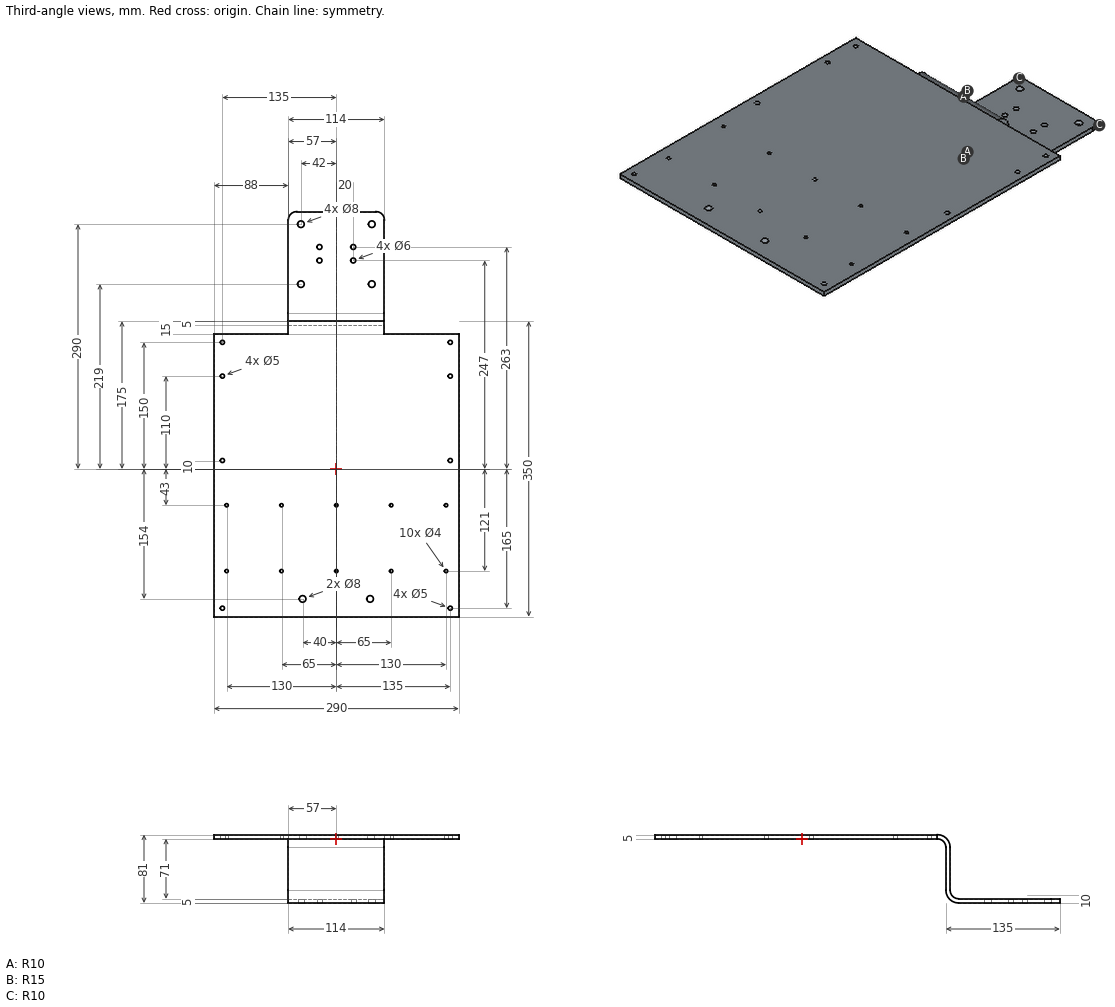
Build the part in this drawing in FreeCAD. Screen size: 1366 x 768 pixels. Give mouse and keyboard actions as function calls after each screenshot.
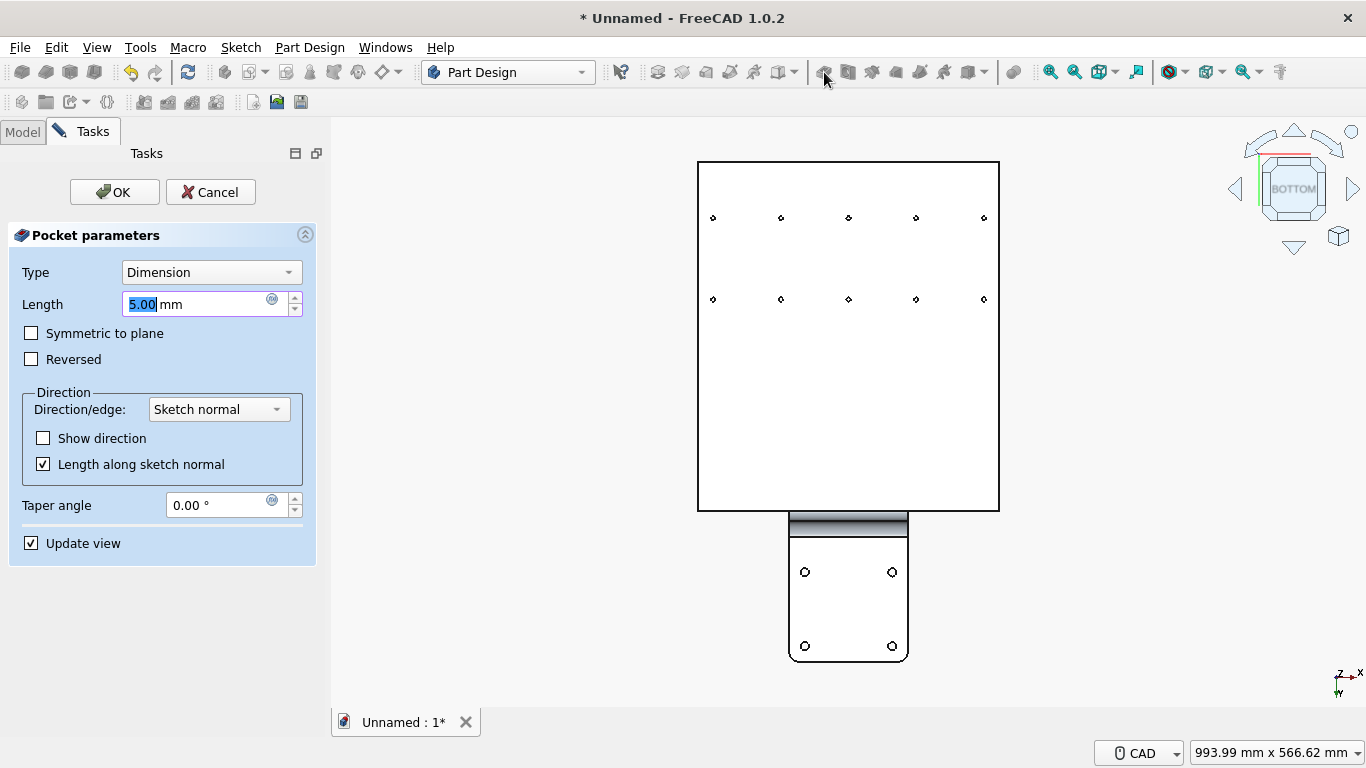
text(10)
key(Tab)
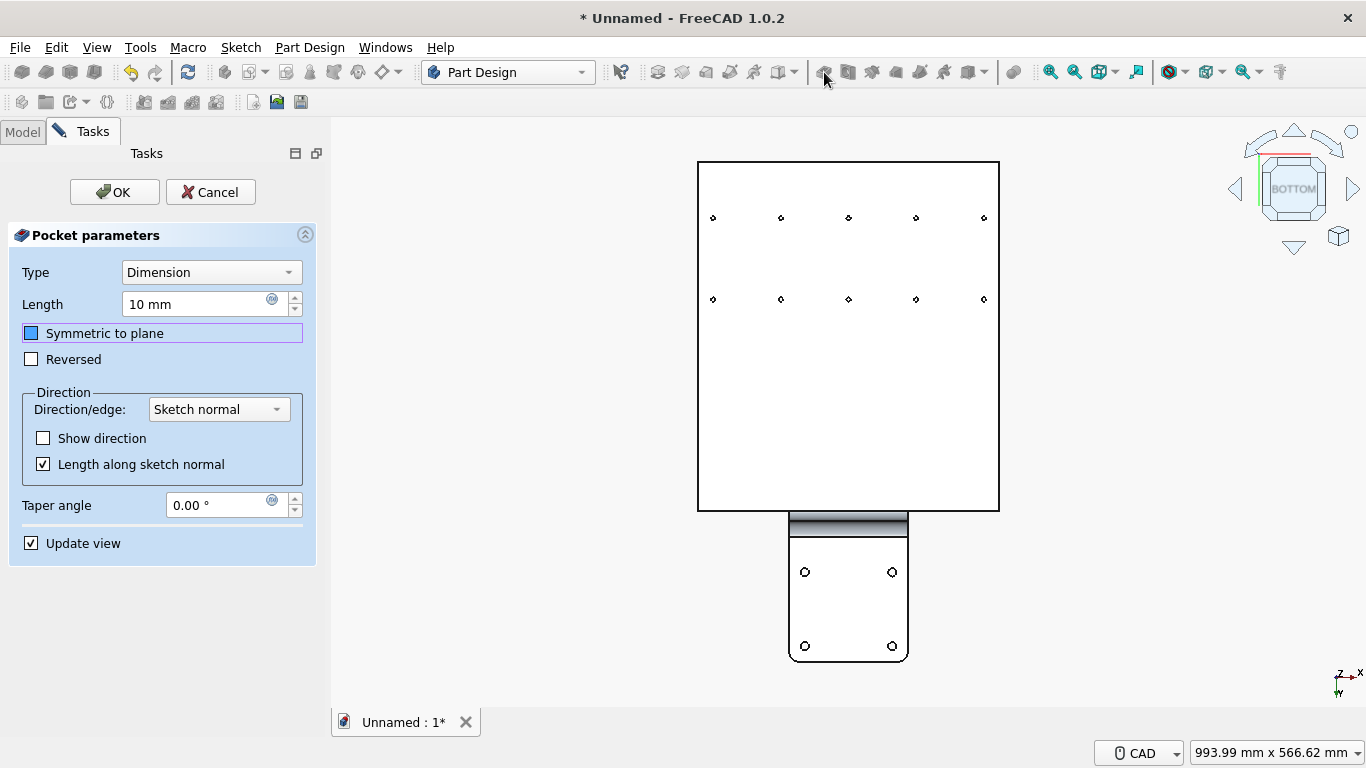
click(115, 192)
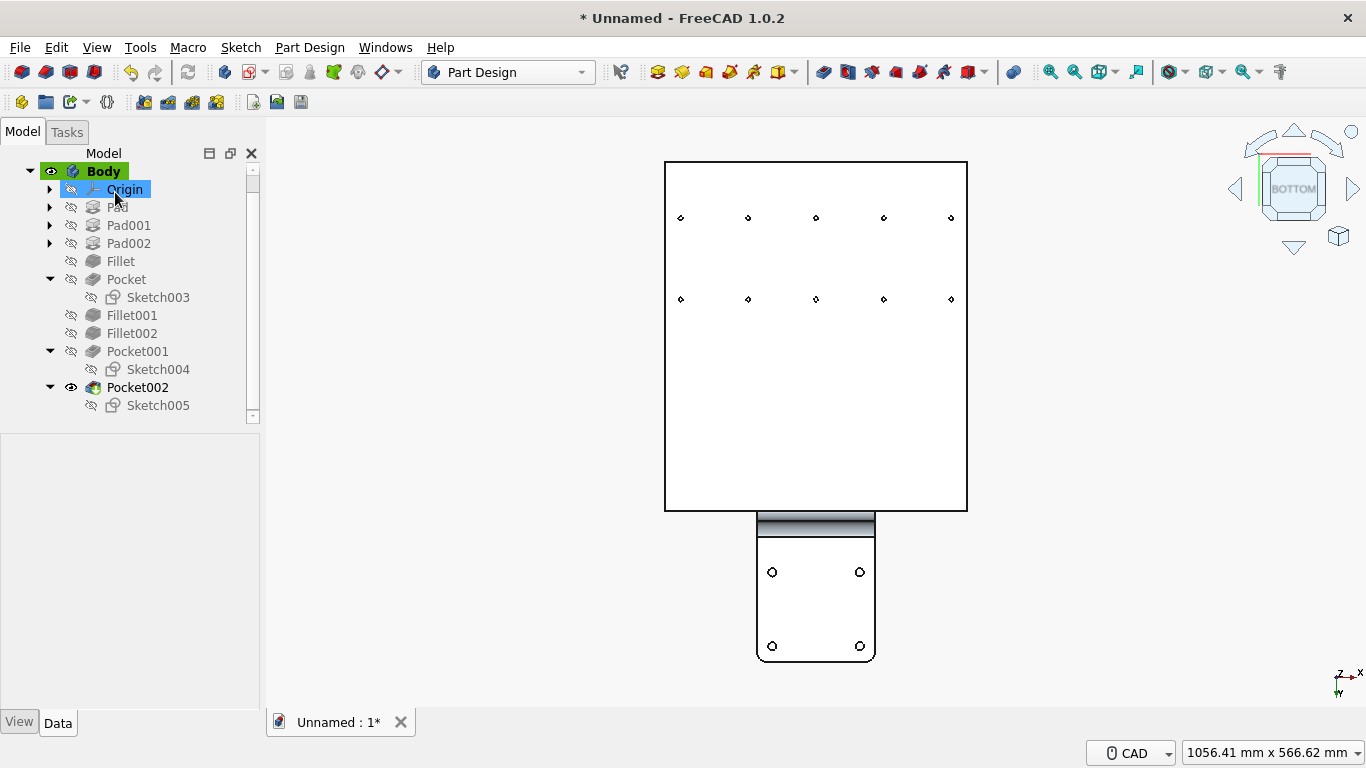
click(816, 598)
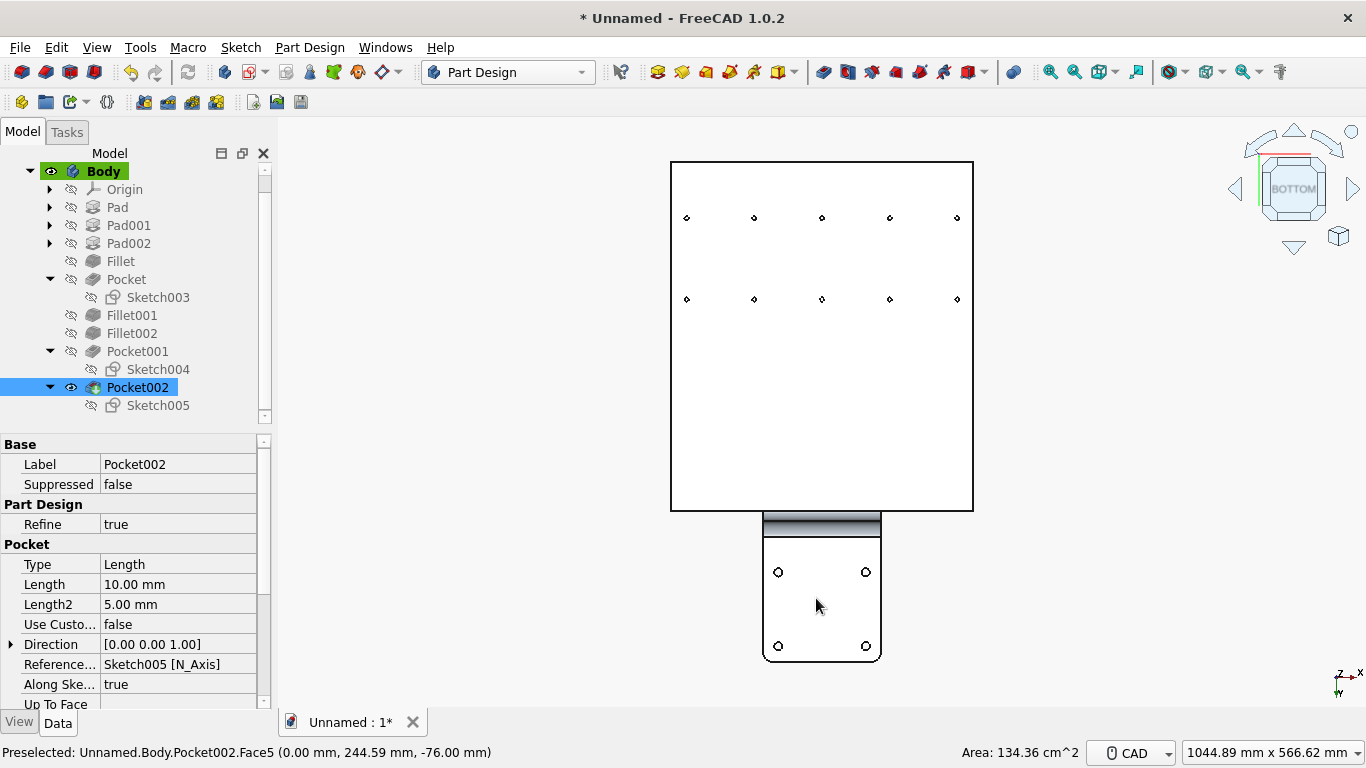
click(250, 72)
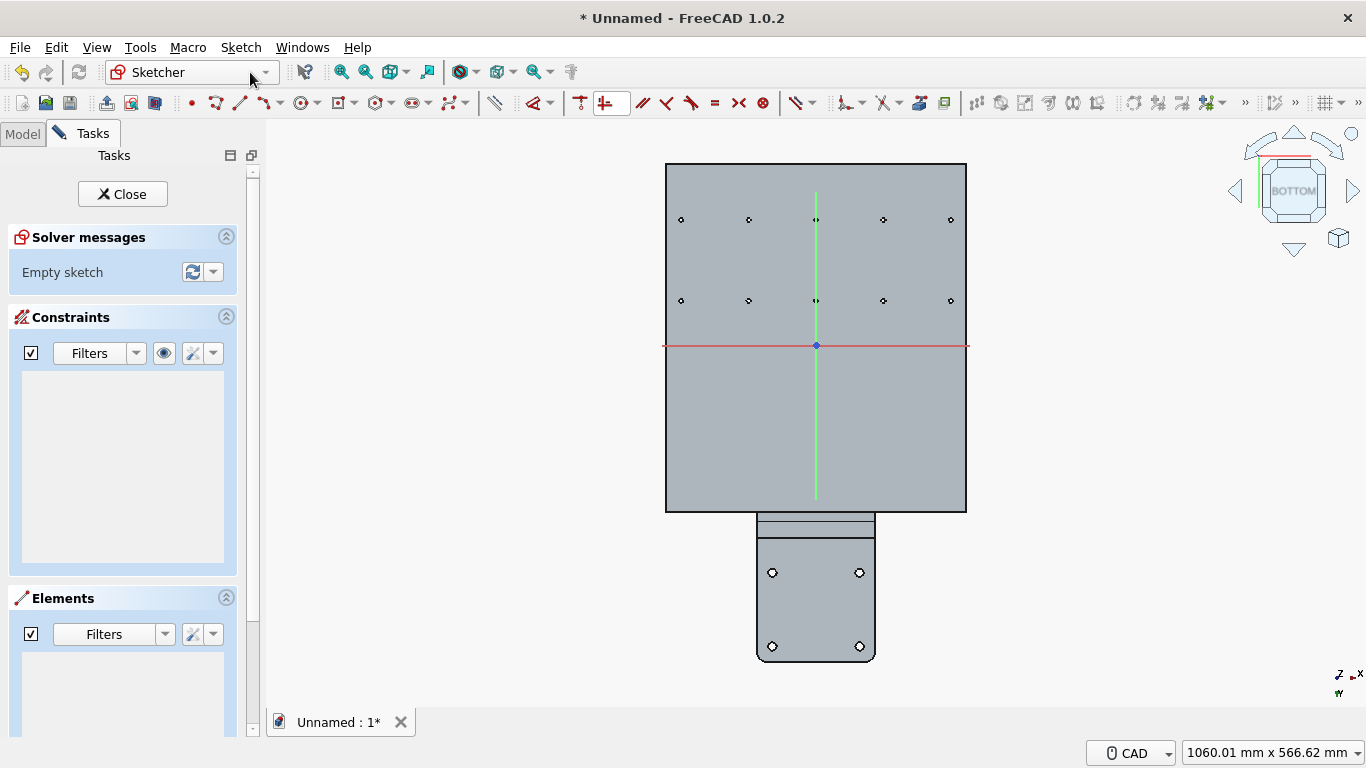
scroll(821, 626, up, 13)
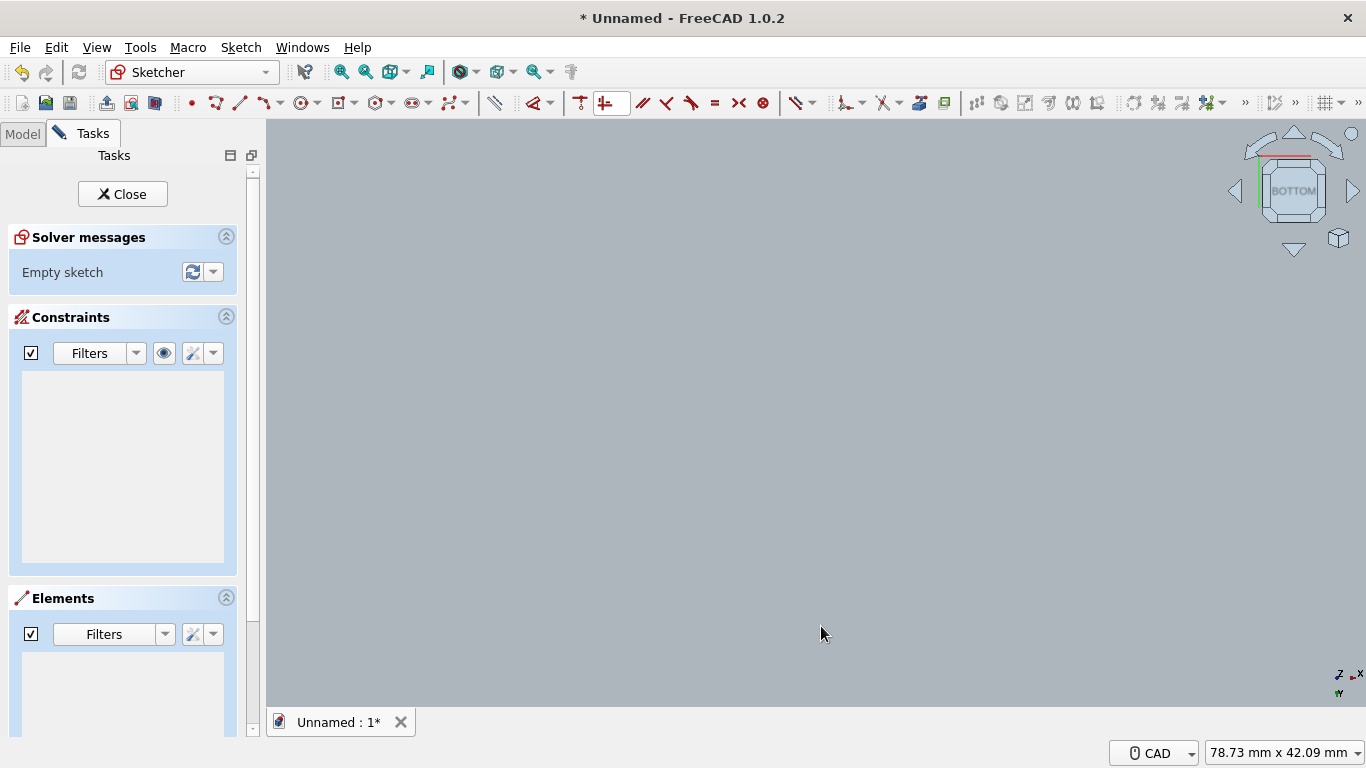
key(g)
key(c)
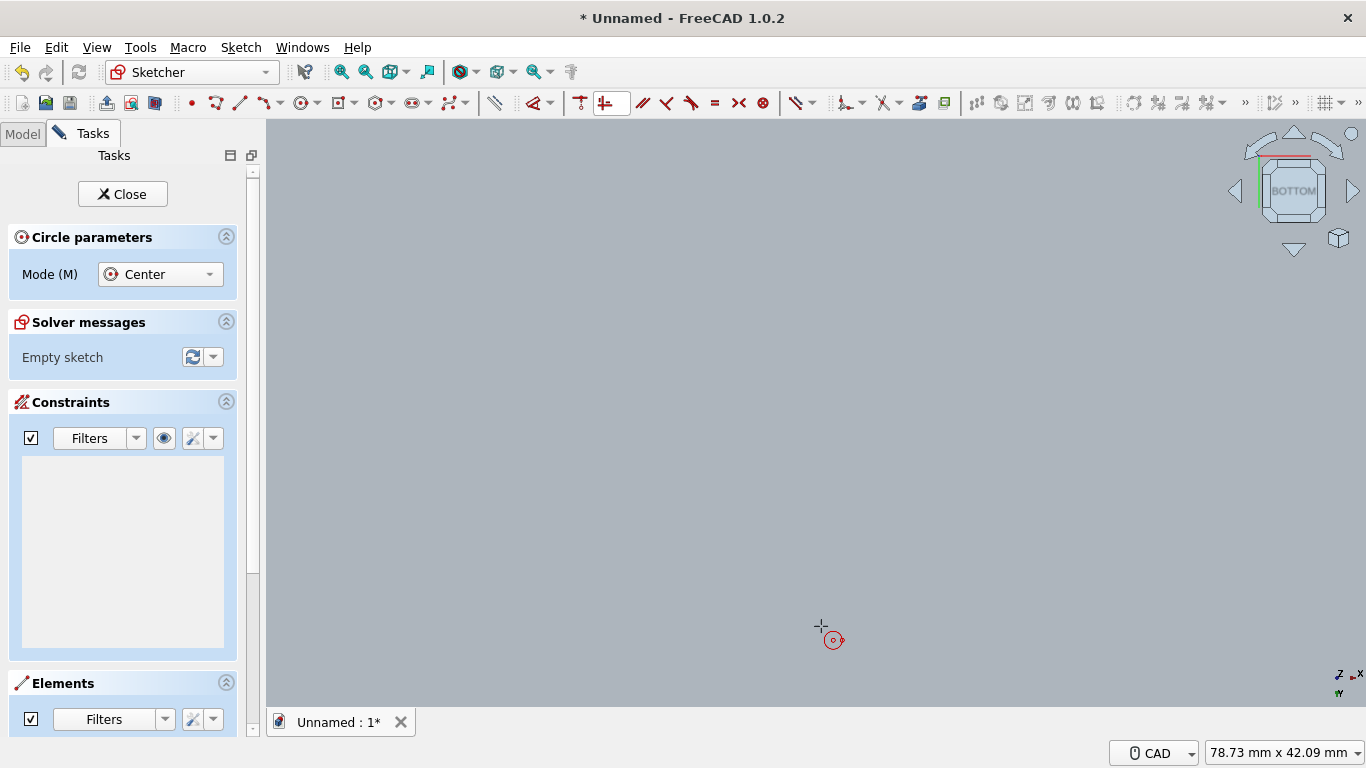
click(1027, 290)
click(1056, 261)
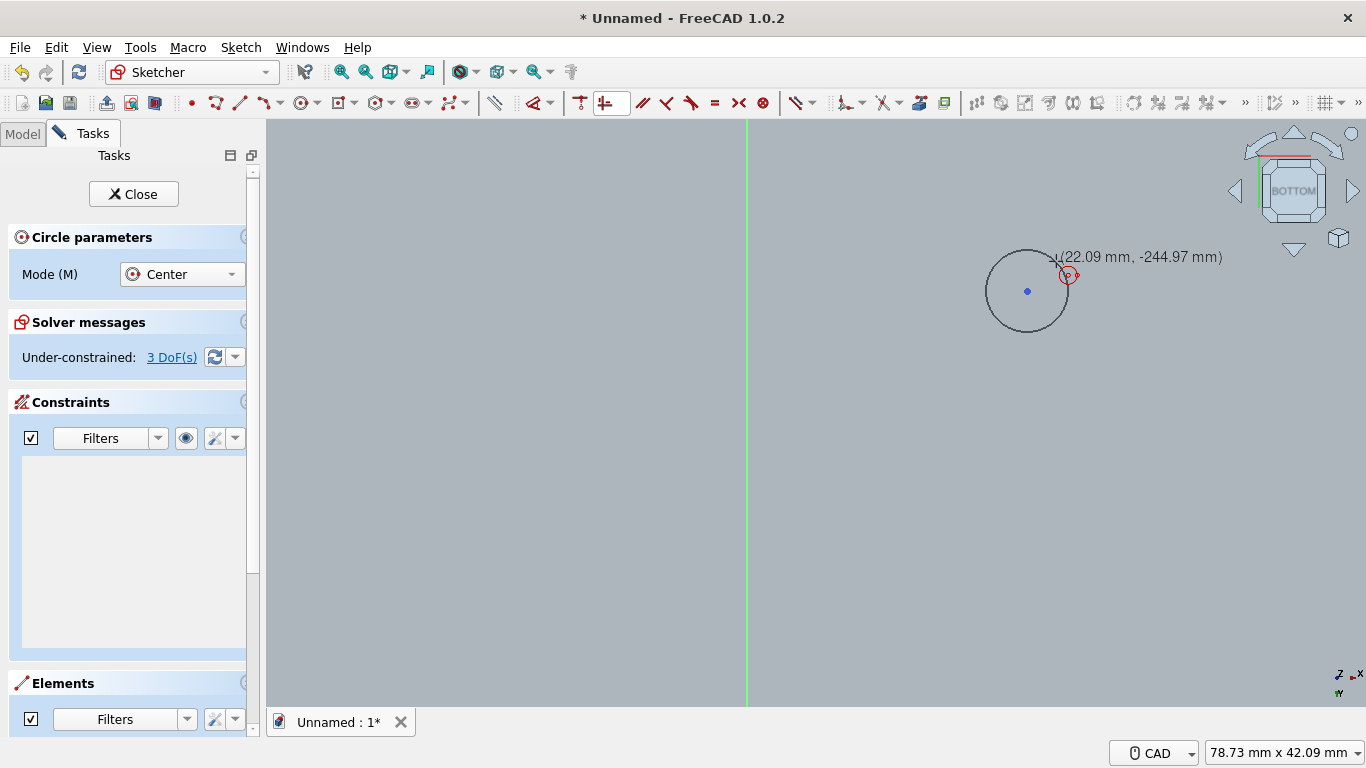
click(1027, 514)
click(1056, 484)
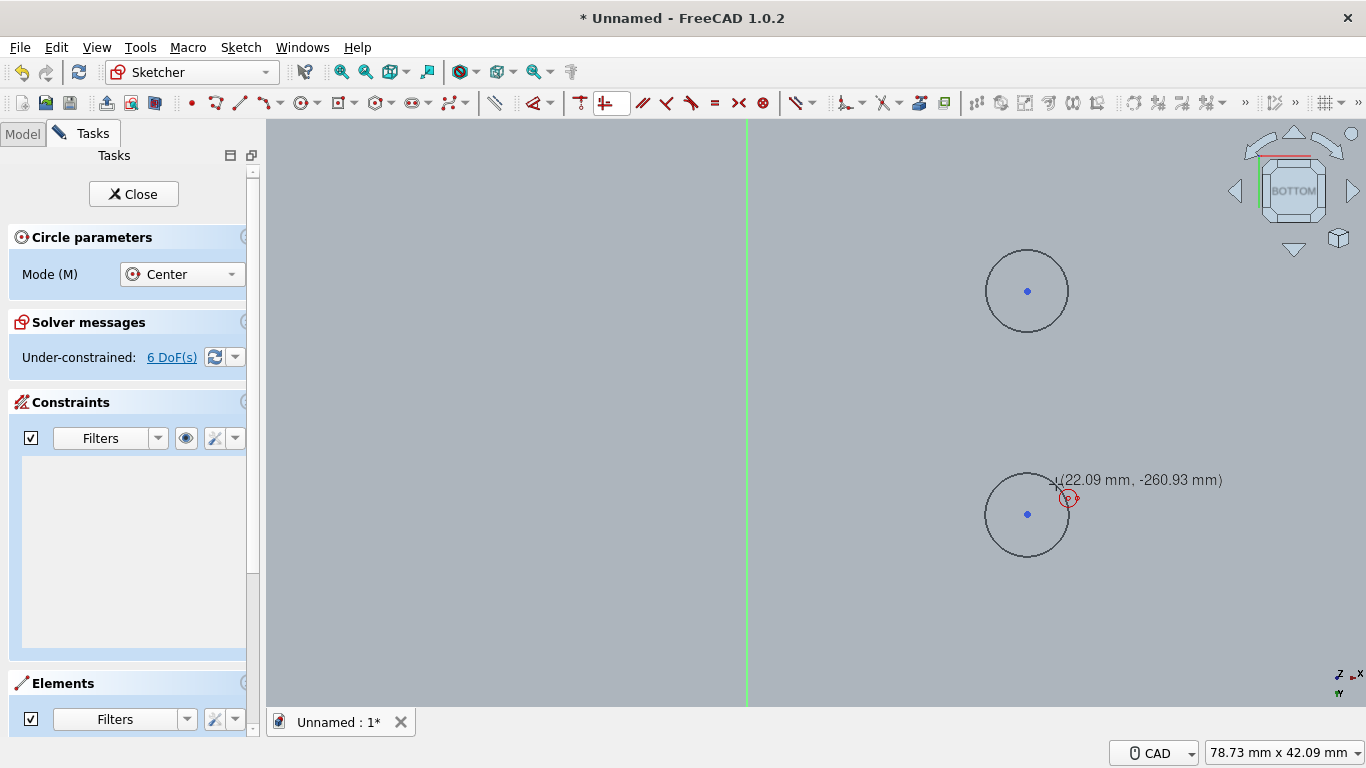
click(468, 514)
click(498, 484)